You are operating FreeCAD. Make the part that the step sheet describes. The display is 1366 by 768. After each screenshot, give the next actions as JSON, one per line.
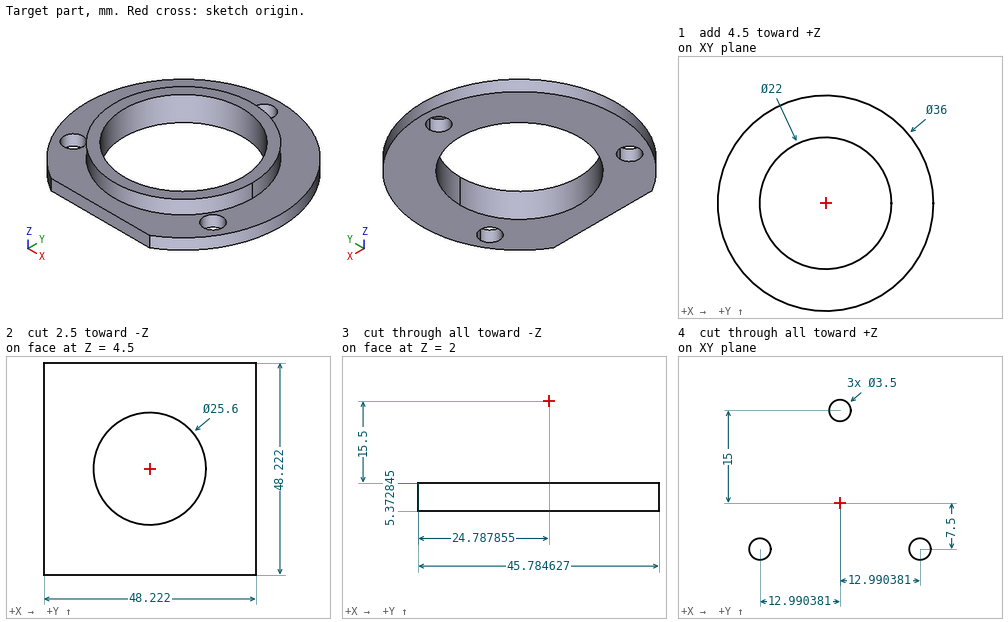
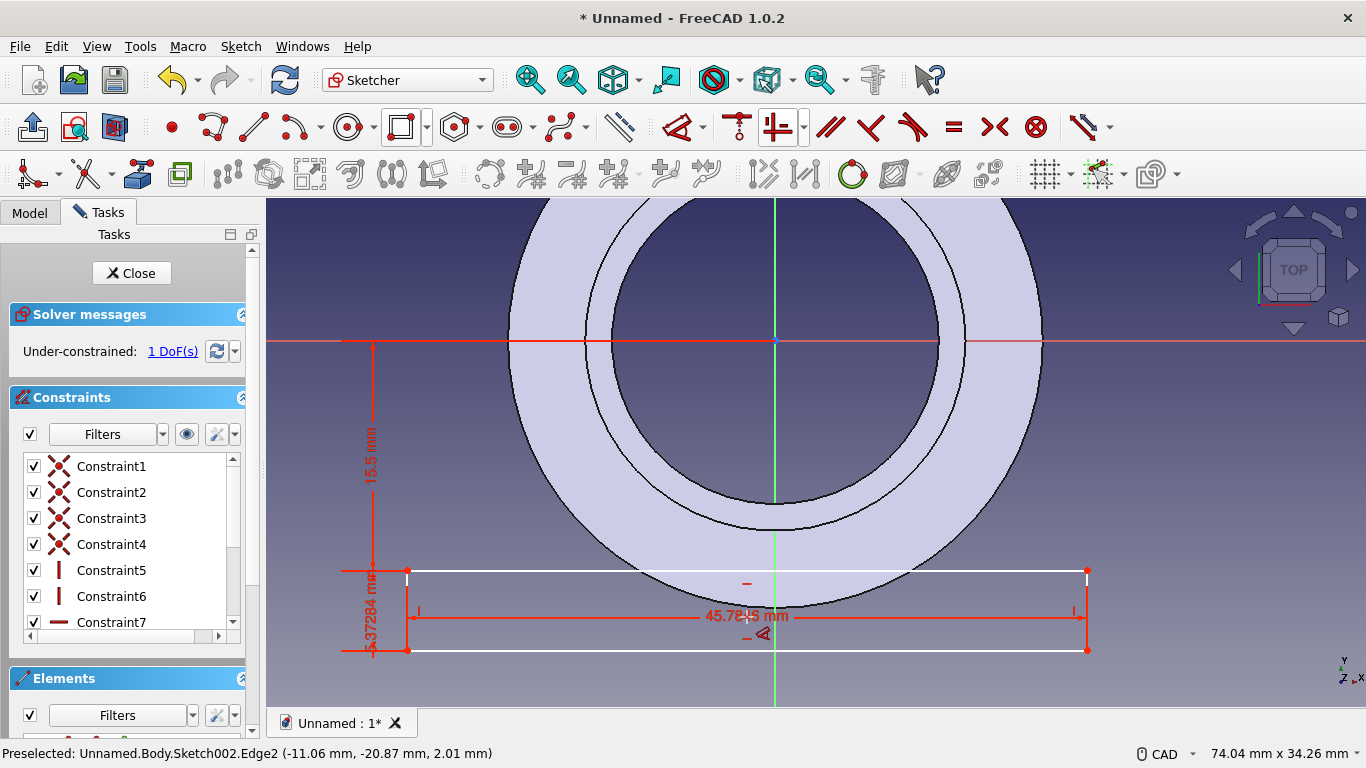
{"action": "left_click", "coordinate": [407, 571]}
{"action": "left_click", "coordinate": [591, 307]}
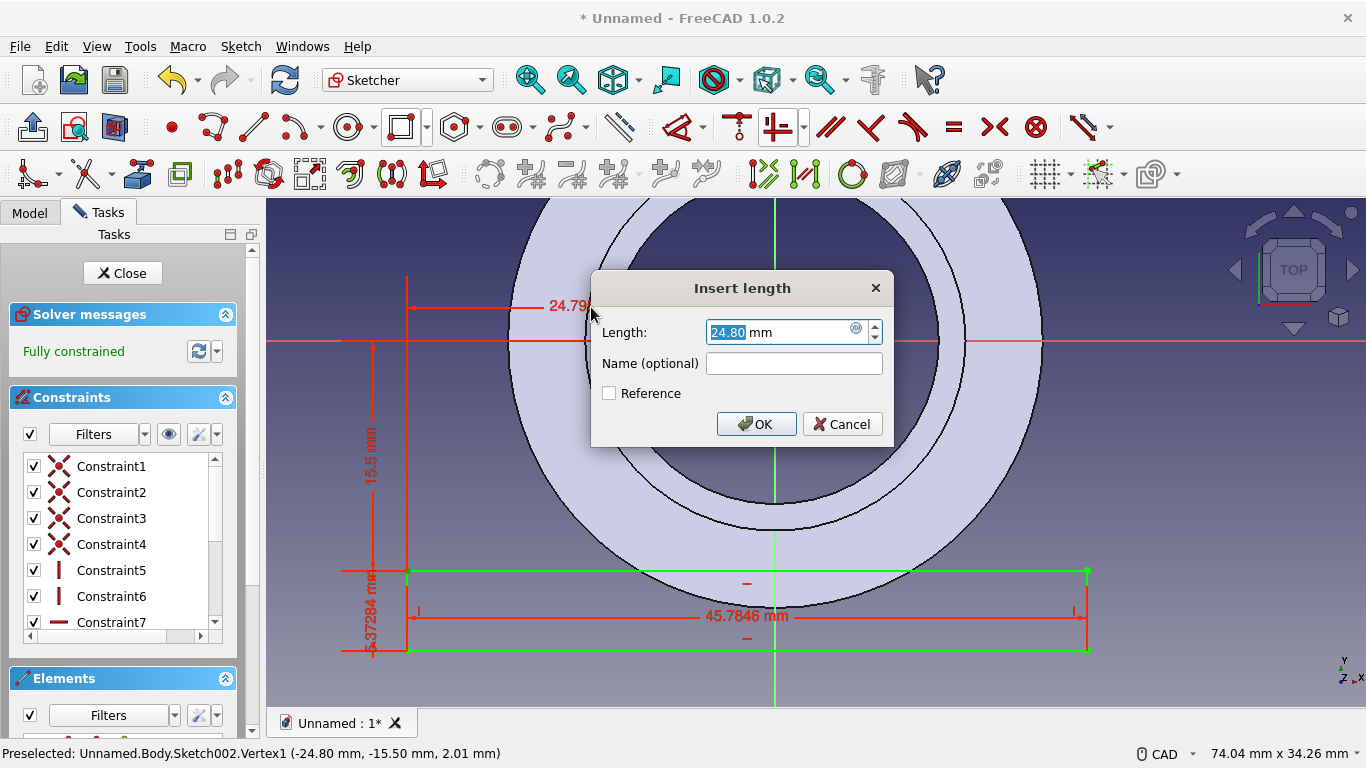
{"action": "type", "text": "24.787855"}
{"action": "key", "text": "Return"}
{"action": "key", "text": "Escape"}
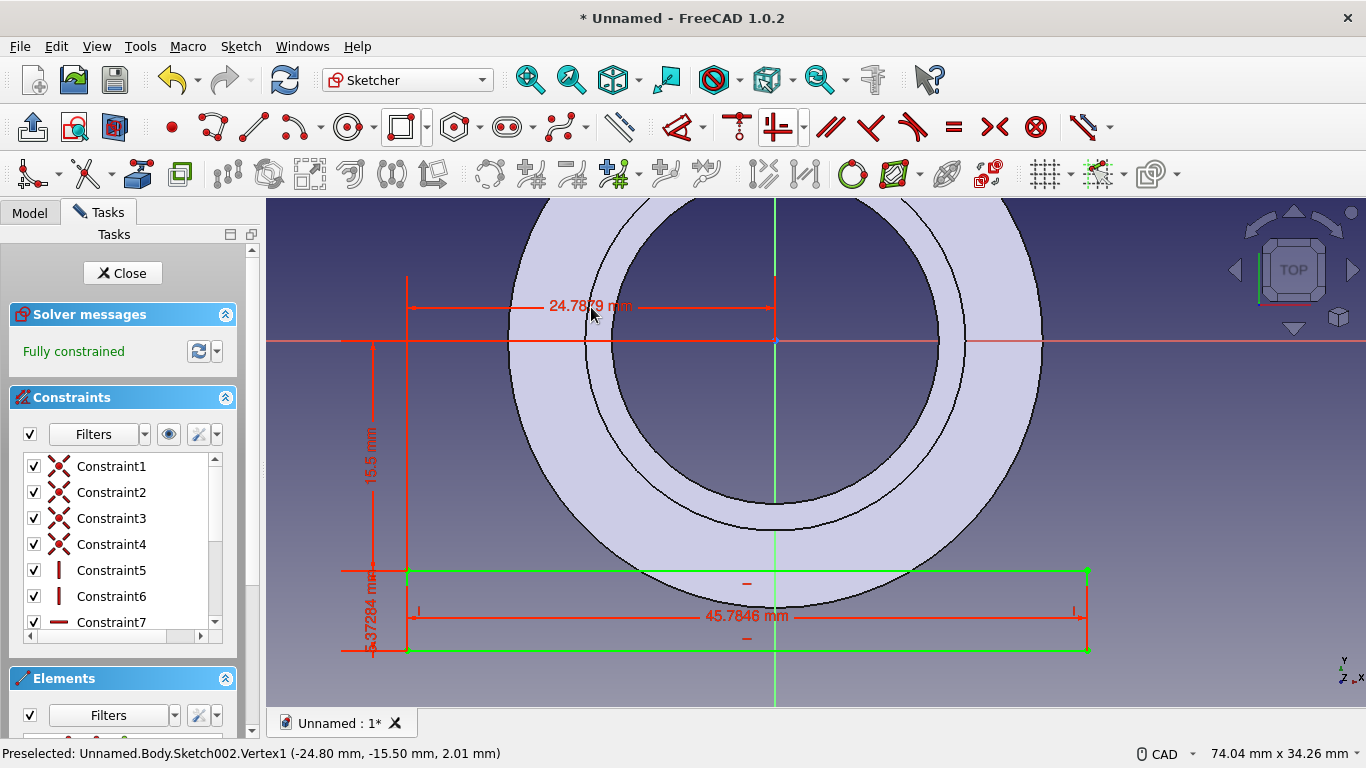
{"action": "left_click", "coordinate": [123, 273]}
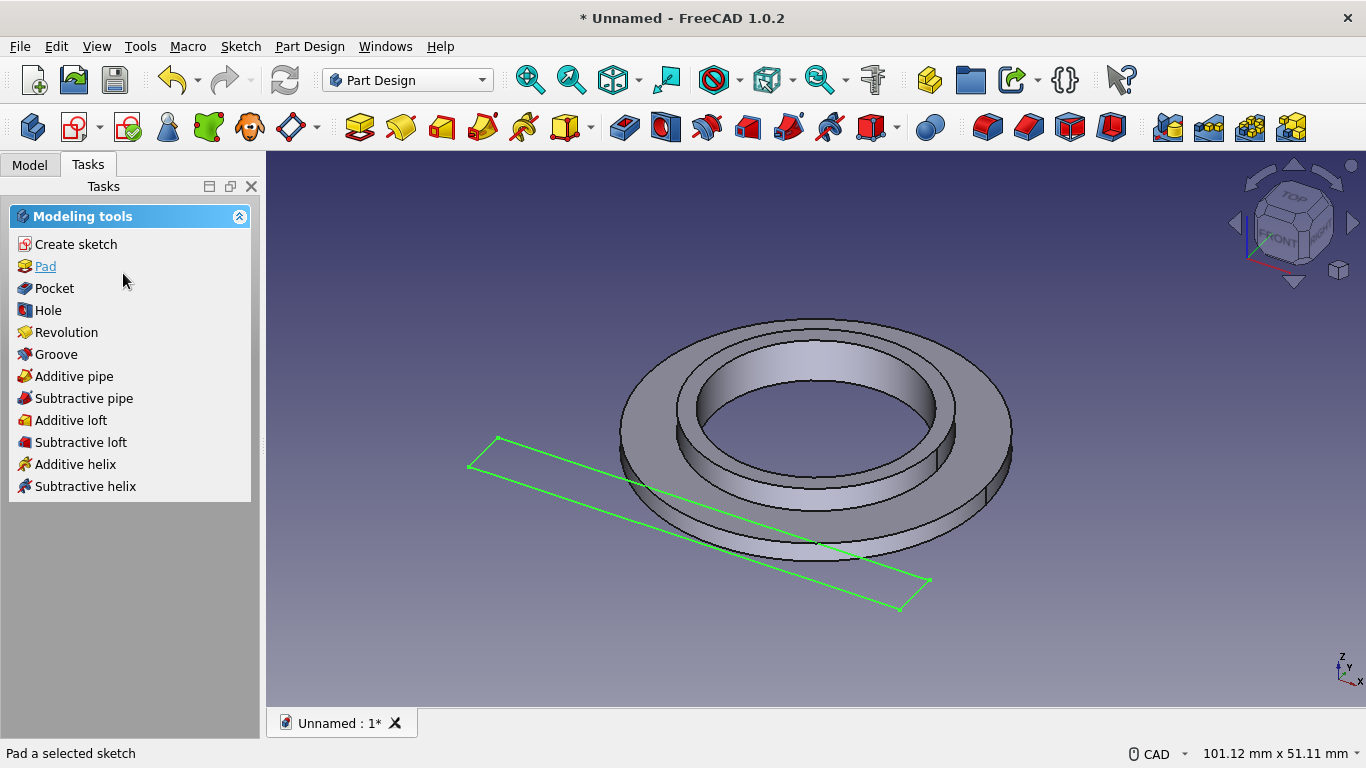
{"action": "left_click", "coordinate": [625, 128]}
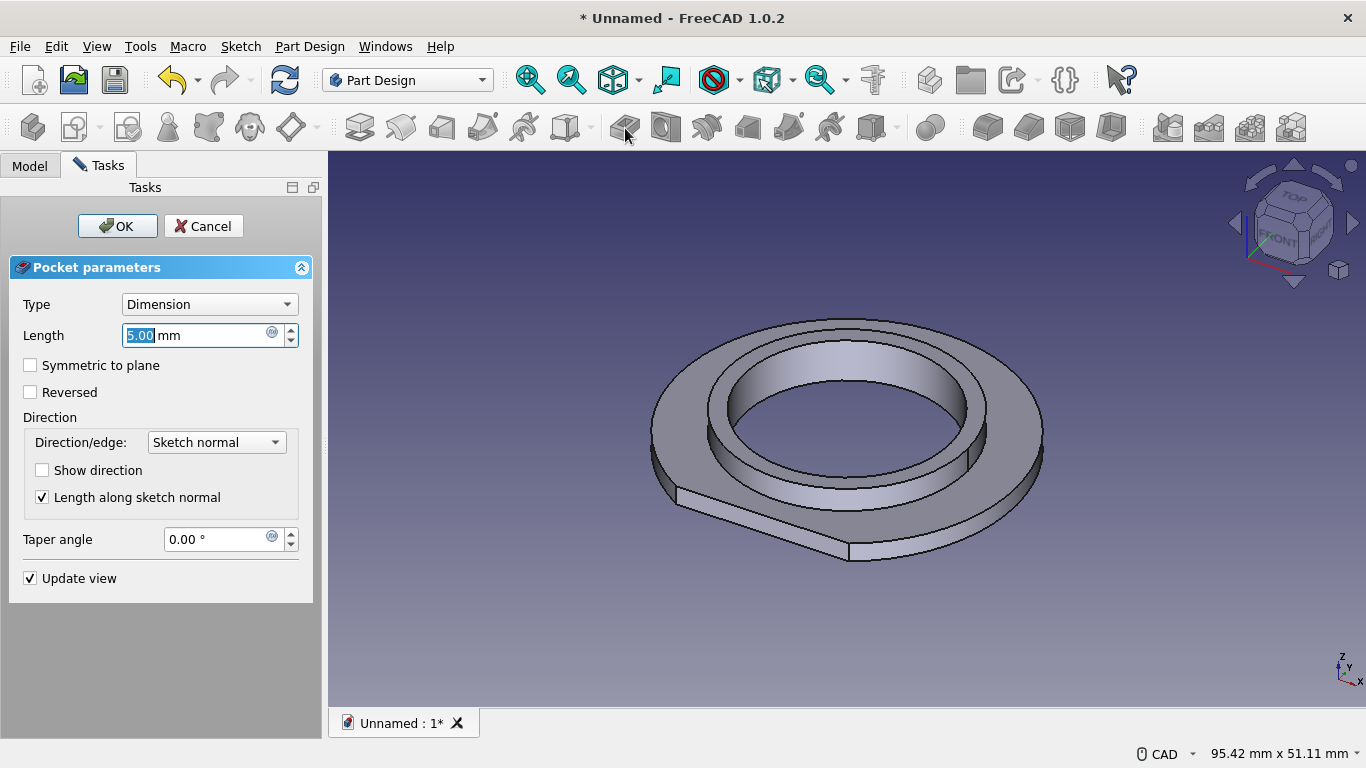
{"action": "left_click", "coordinate": [210, 304]}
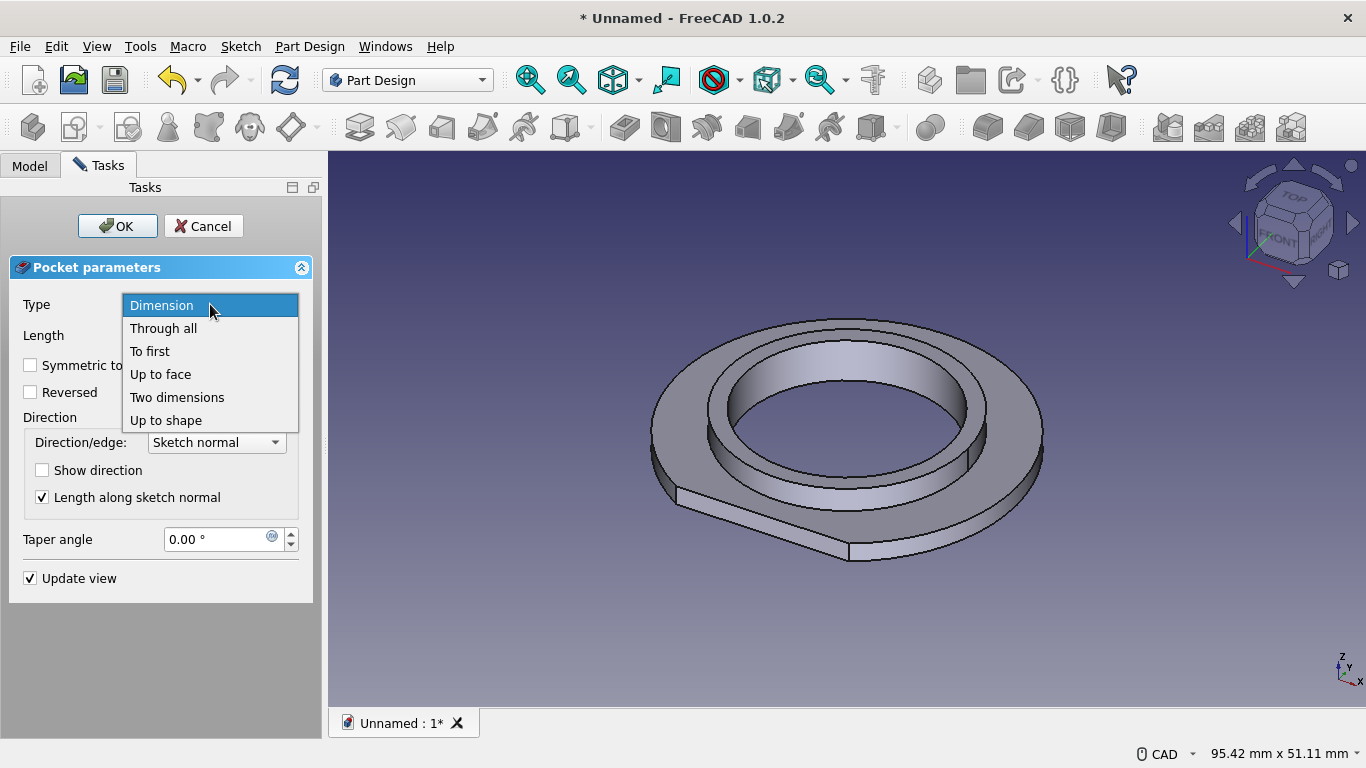
{"action": "left_click", "coordinate": [208, 328]}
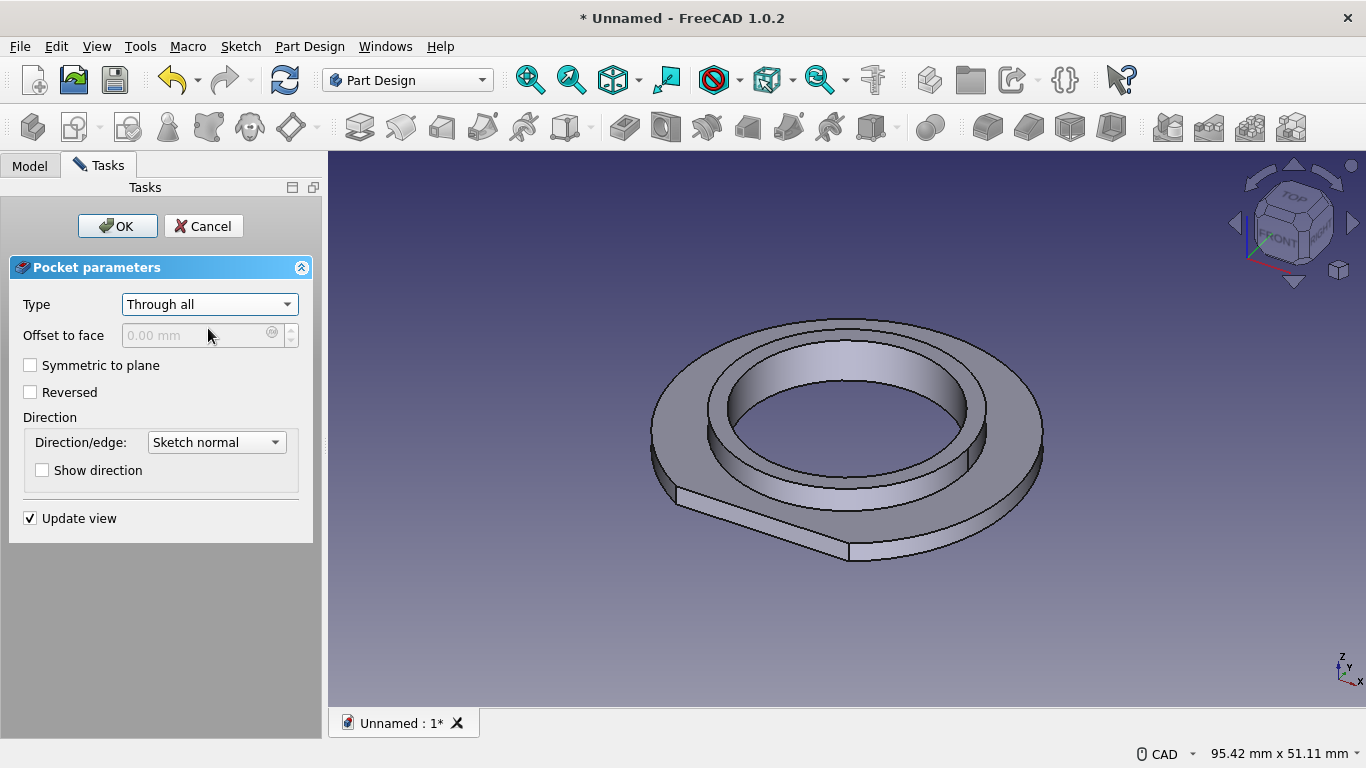
{"action": "left_click", "coordinate": [118, 226]}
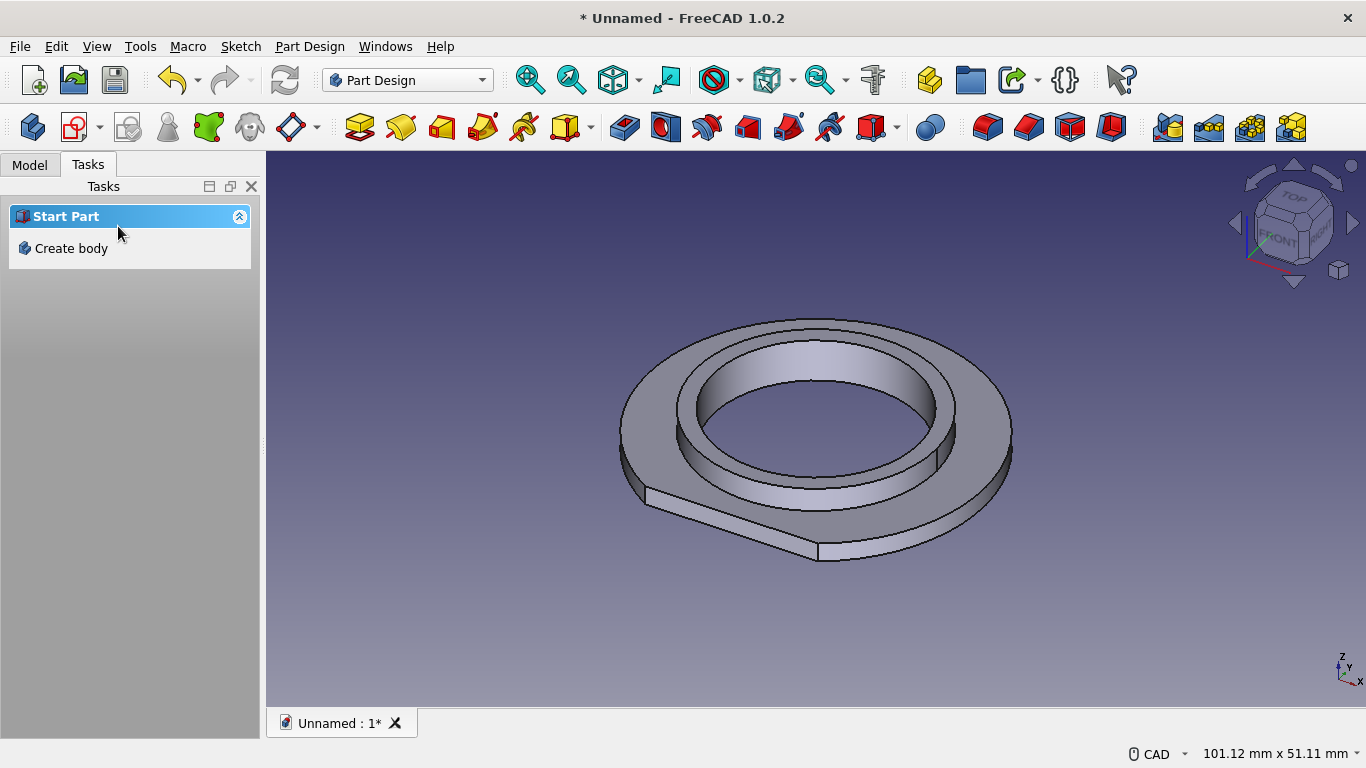
{"action": "left_click", "coordinate": [74, 128]}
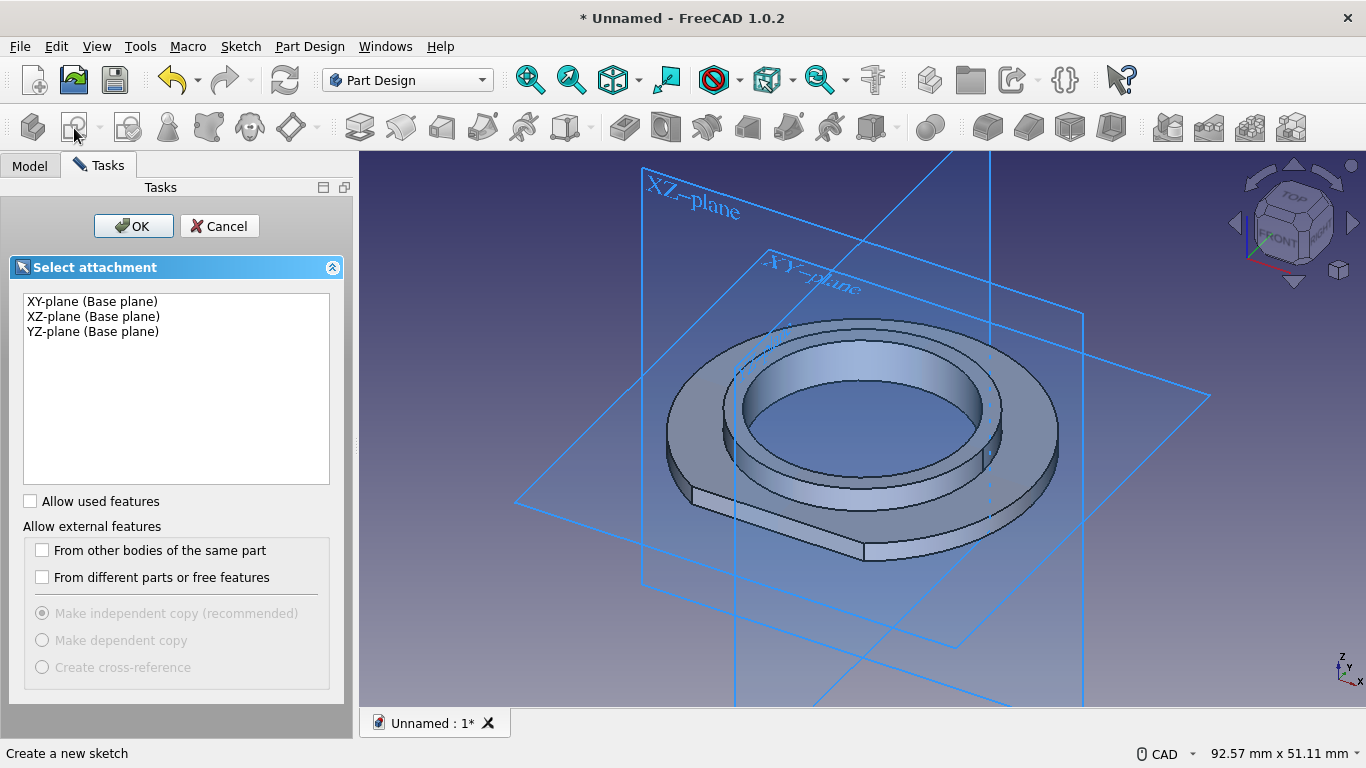
{"action": "left_click", "coordinate": [84, 302]}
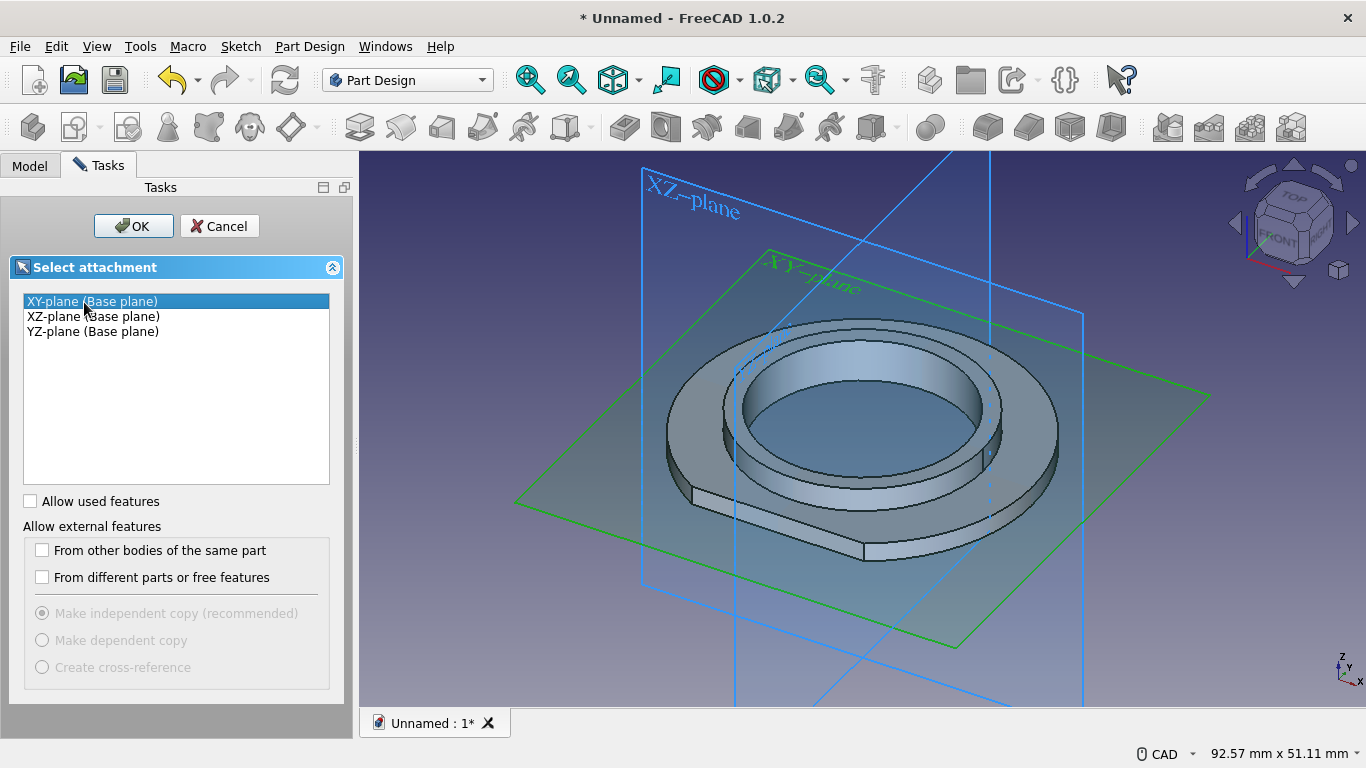
{"action": "left_click", "coordinate": [134, 226]}